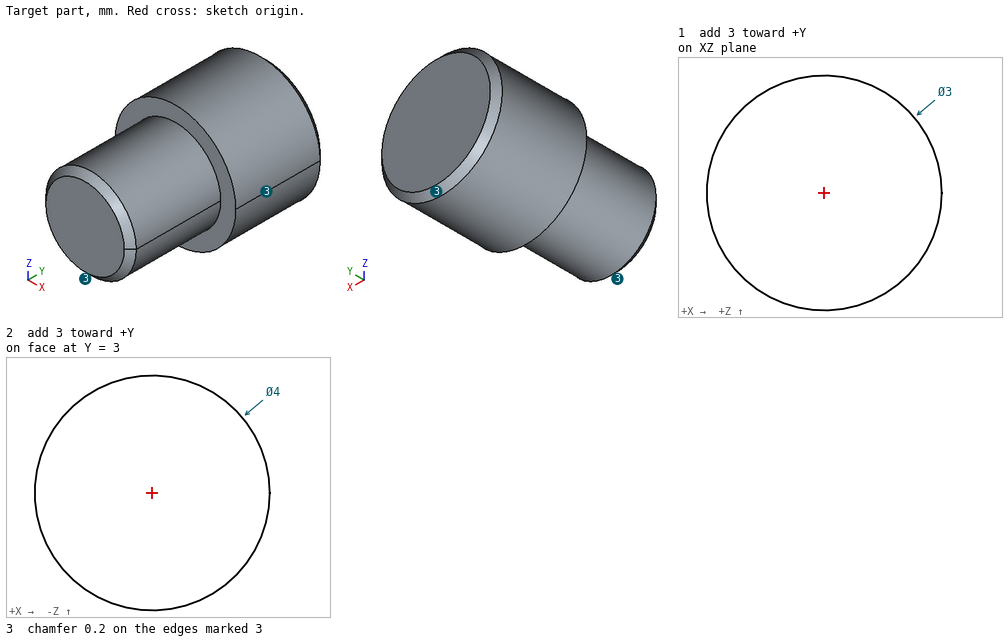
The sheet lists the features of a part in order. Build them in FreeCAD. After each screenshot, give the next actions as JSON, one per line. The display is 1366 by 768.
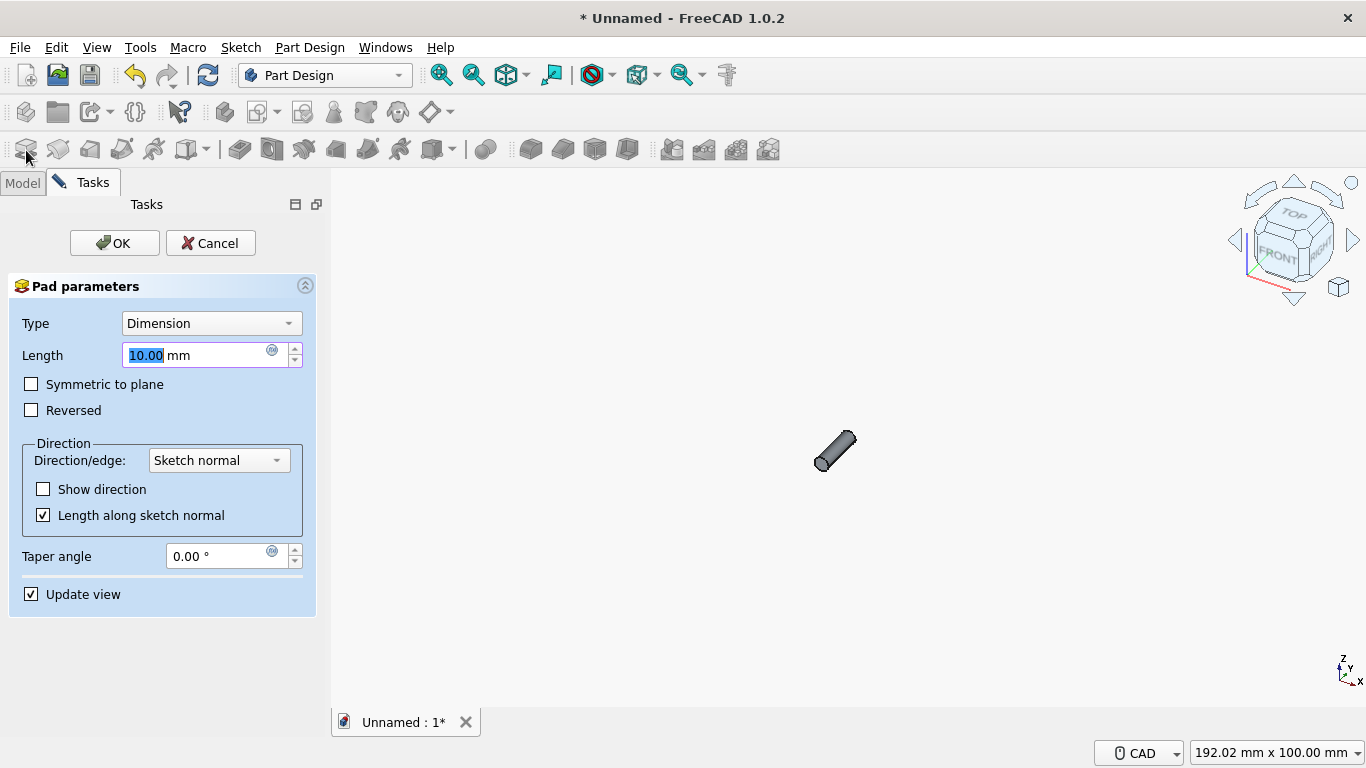
{"action": "type", "text": "3"}
{"action": "key", "text": "Tab"}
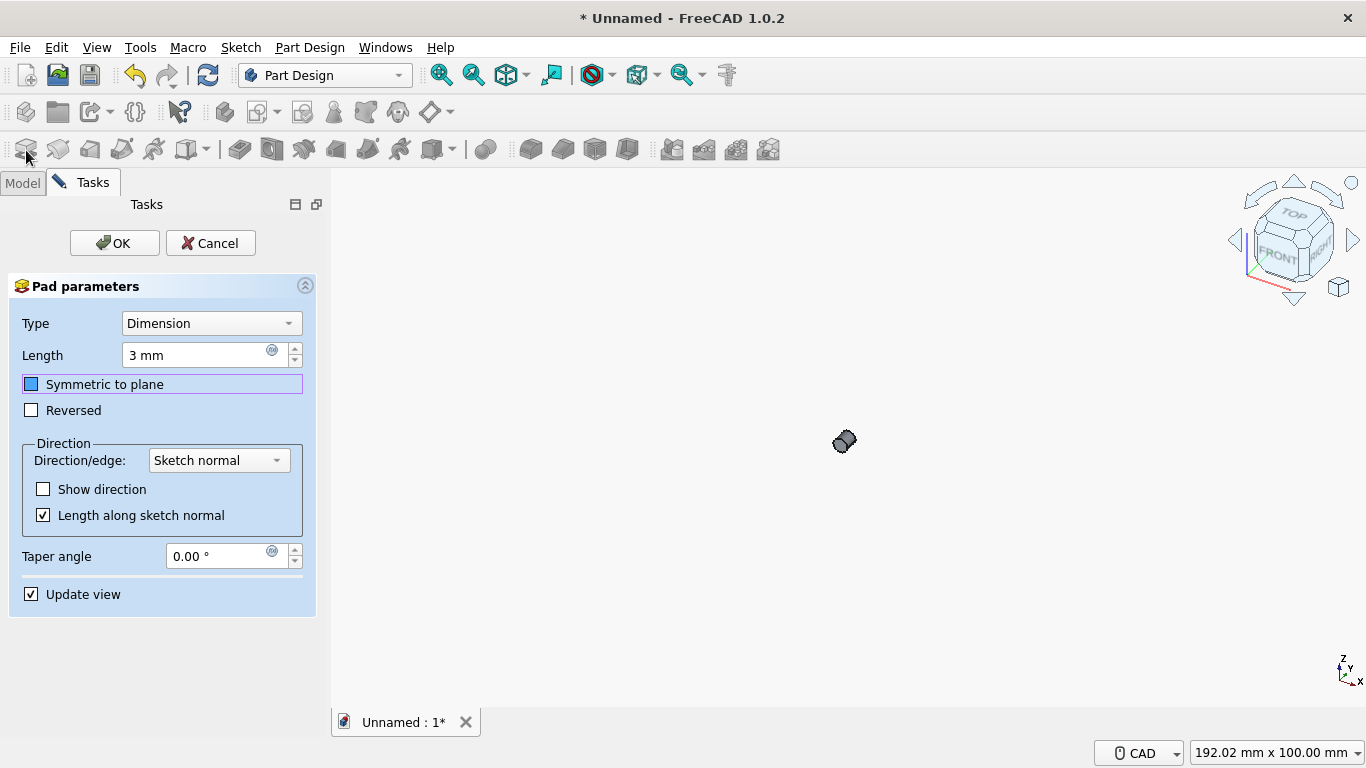
{"action": "left_click", "coordinate": [30, 410]}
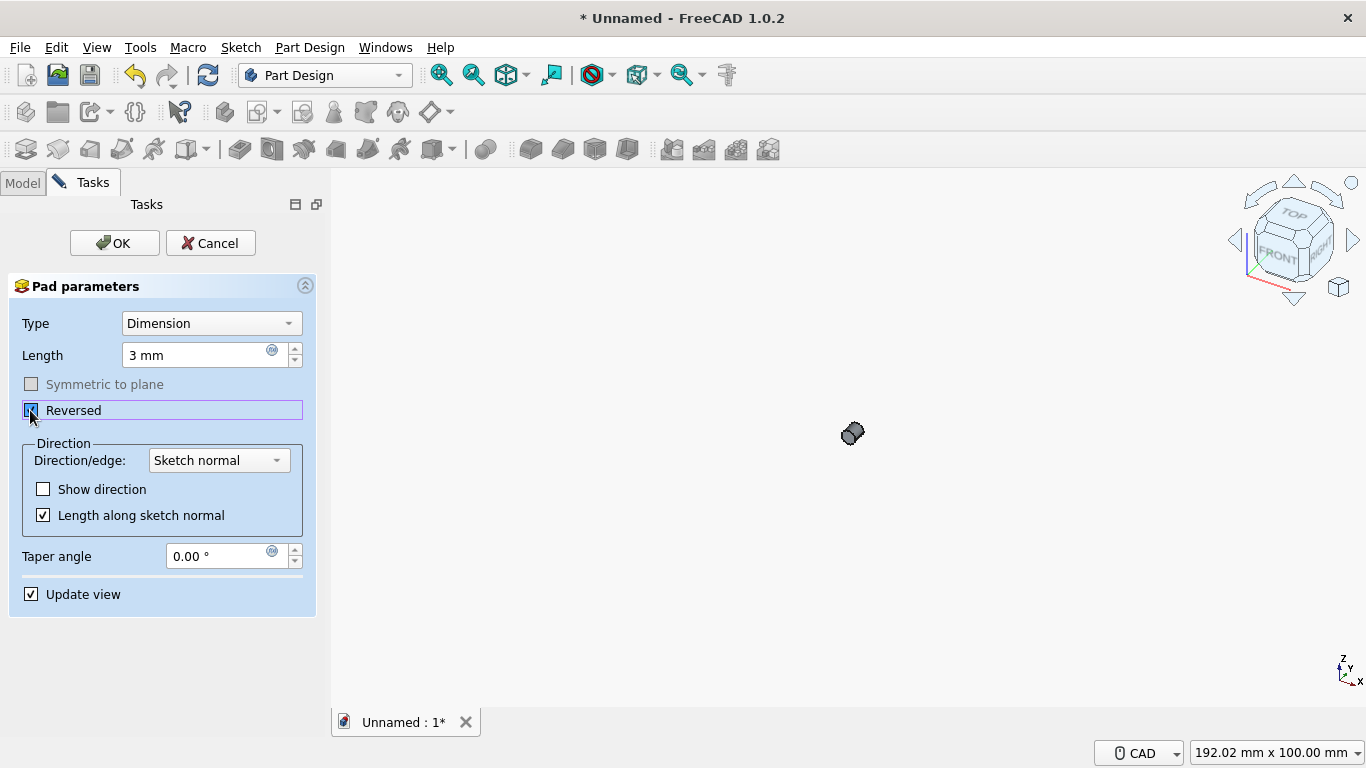
{"action": "left_click", "coordinate": [115, 243]}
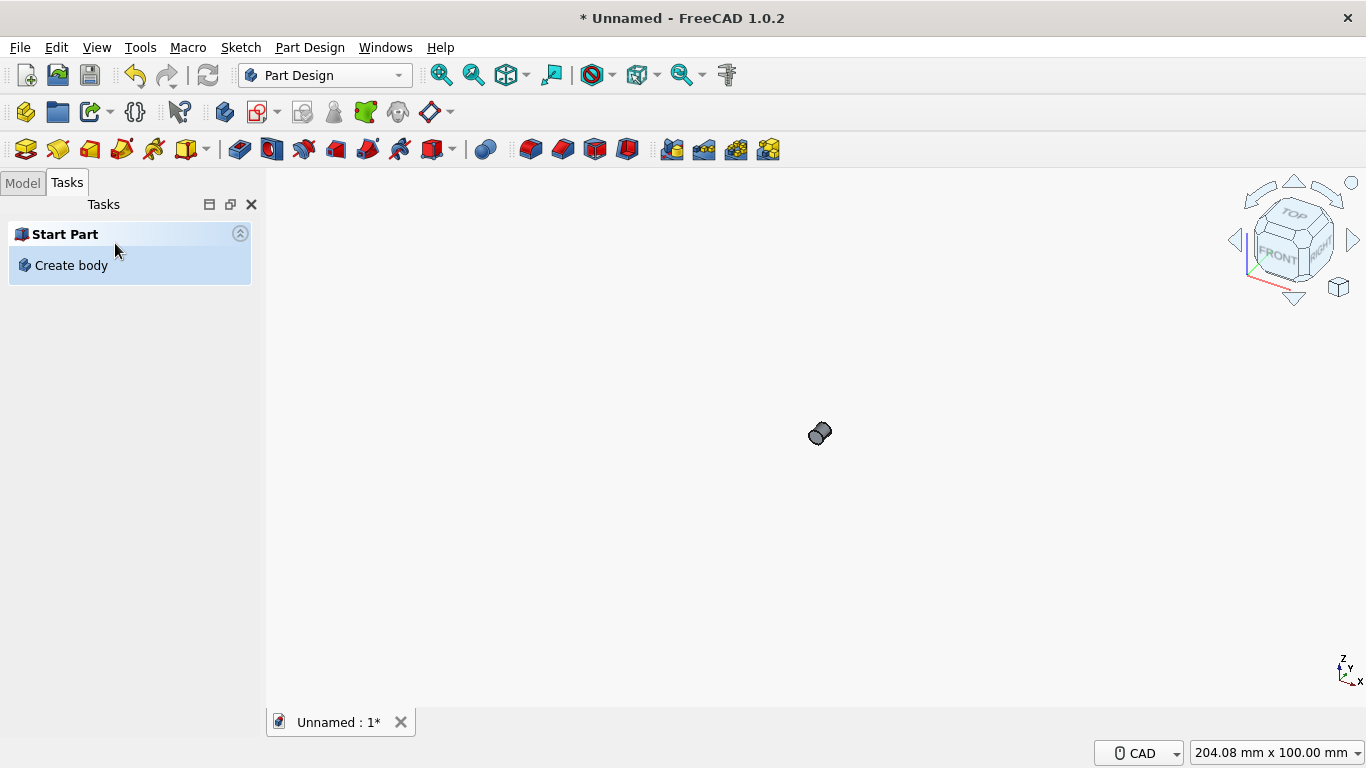
{"action": "left_click", "coordinate": [442, 76]}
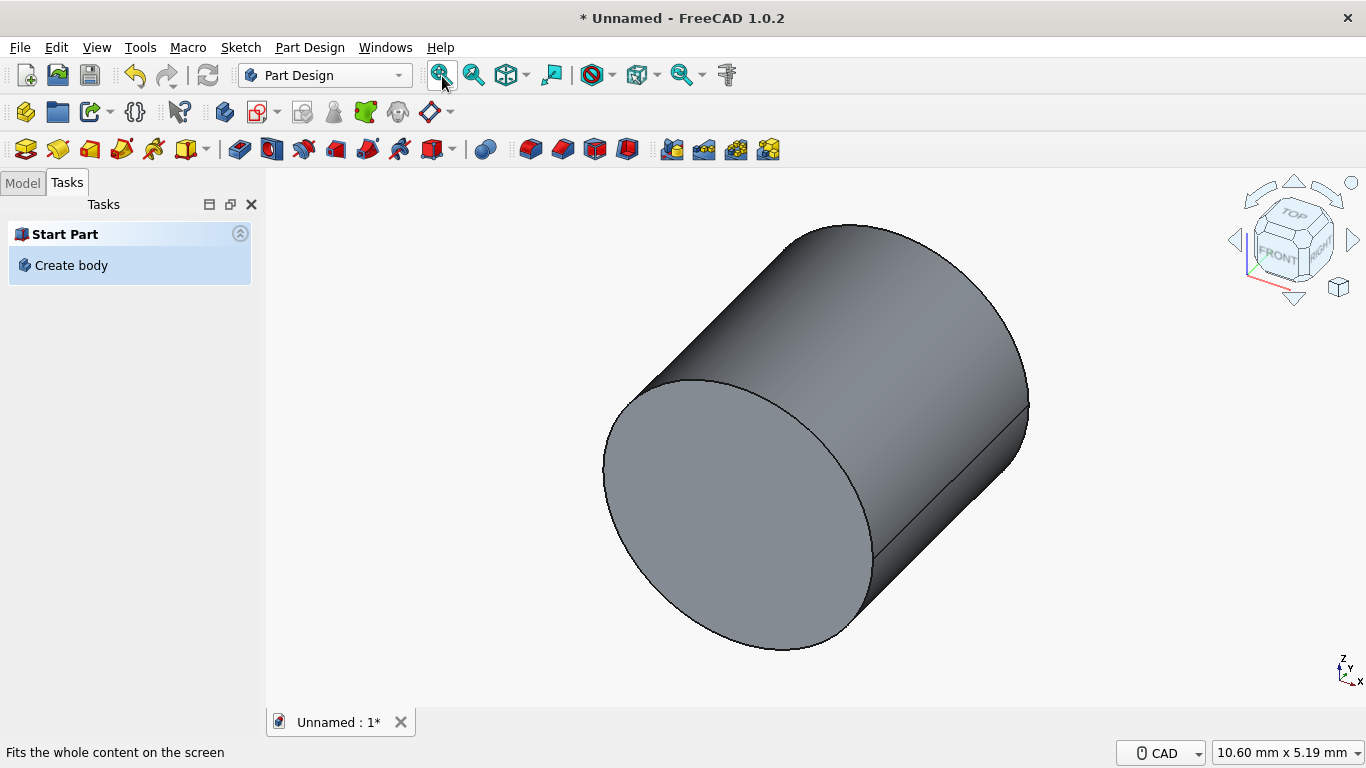
{"action": "key", "text": "4"}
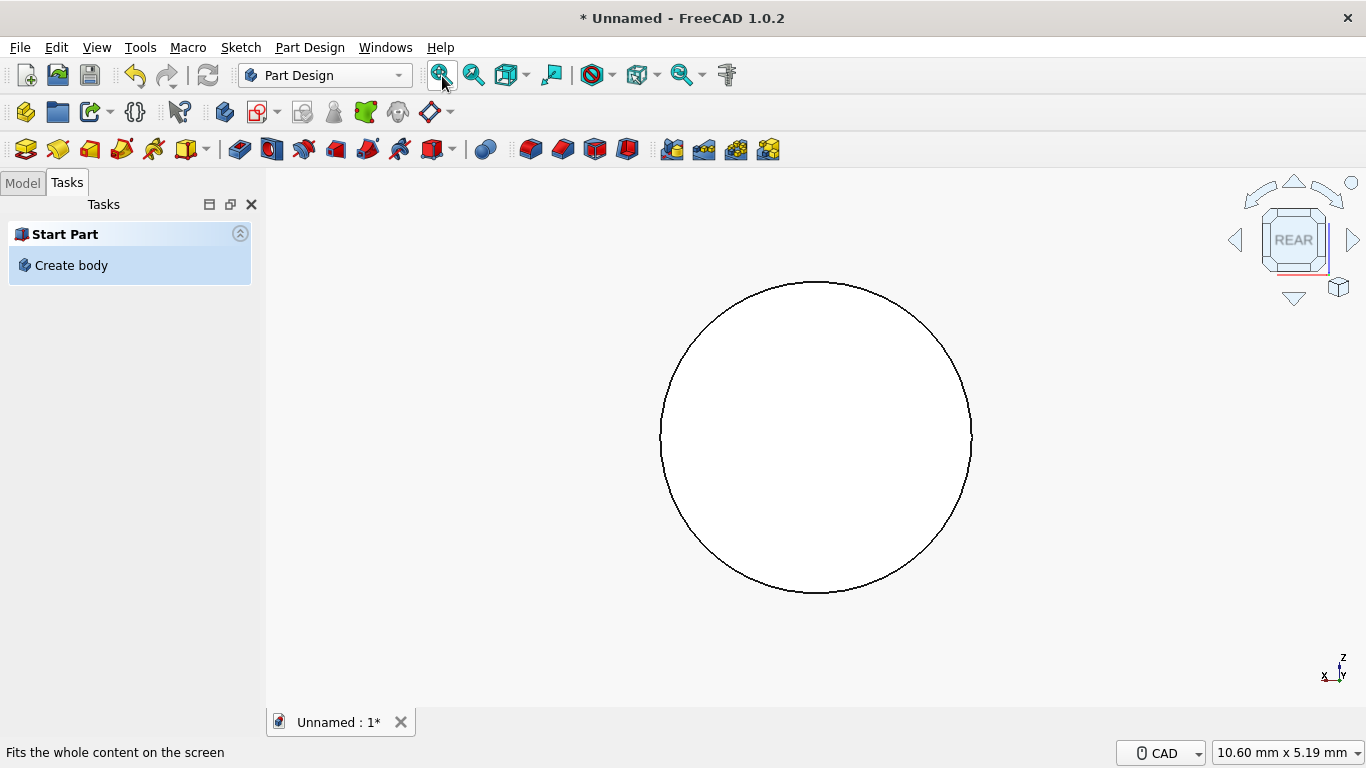
{"action": "left_click", "coordinate": [816, 437]}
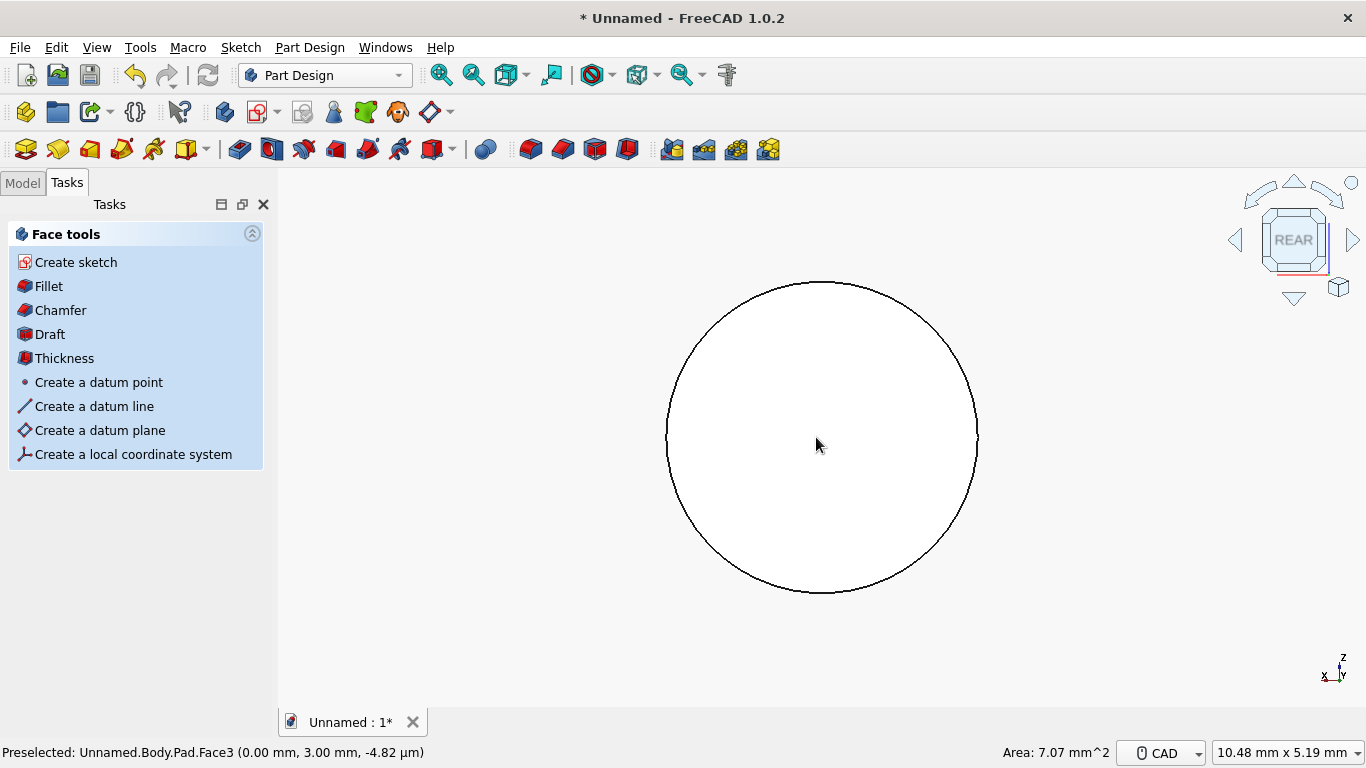
{"action": "left_click", "coordinate": [258, 112]}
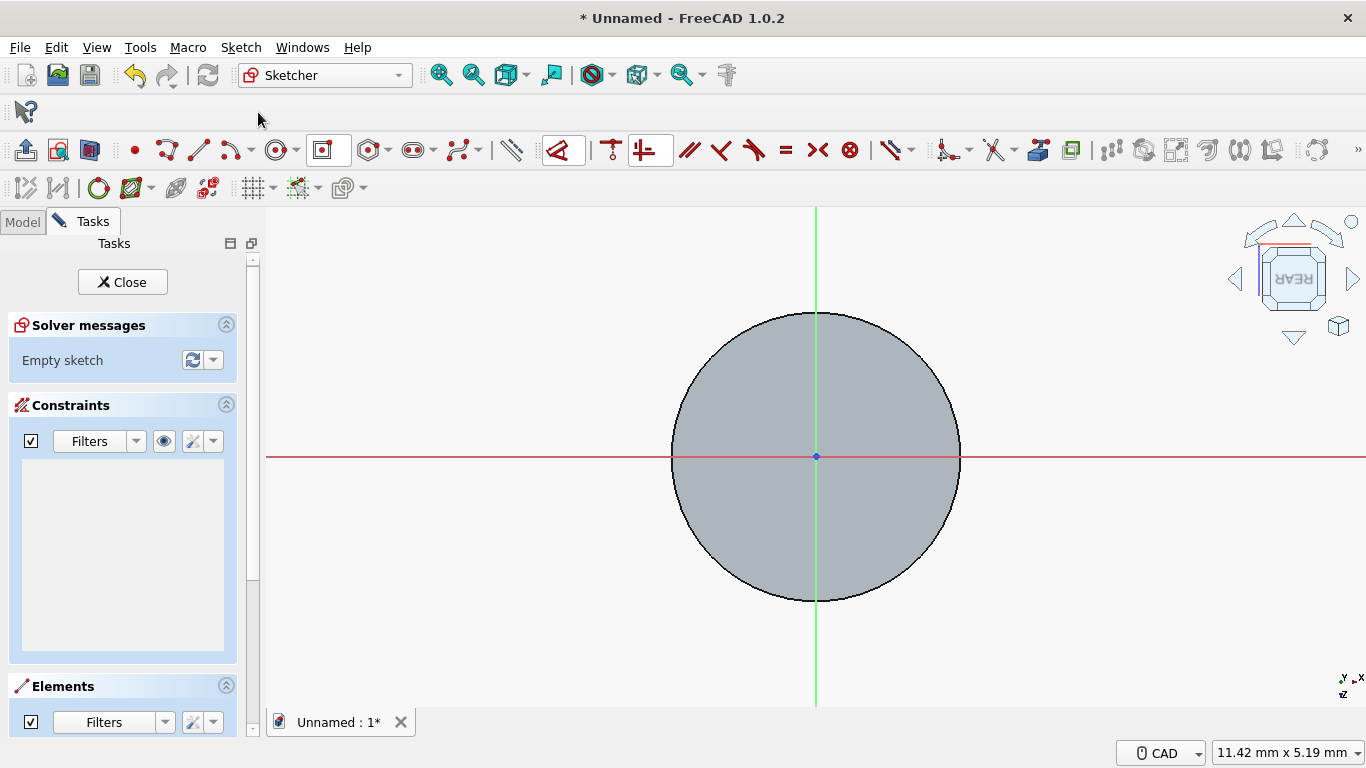
{"action": "key", "text": "g c"}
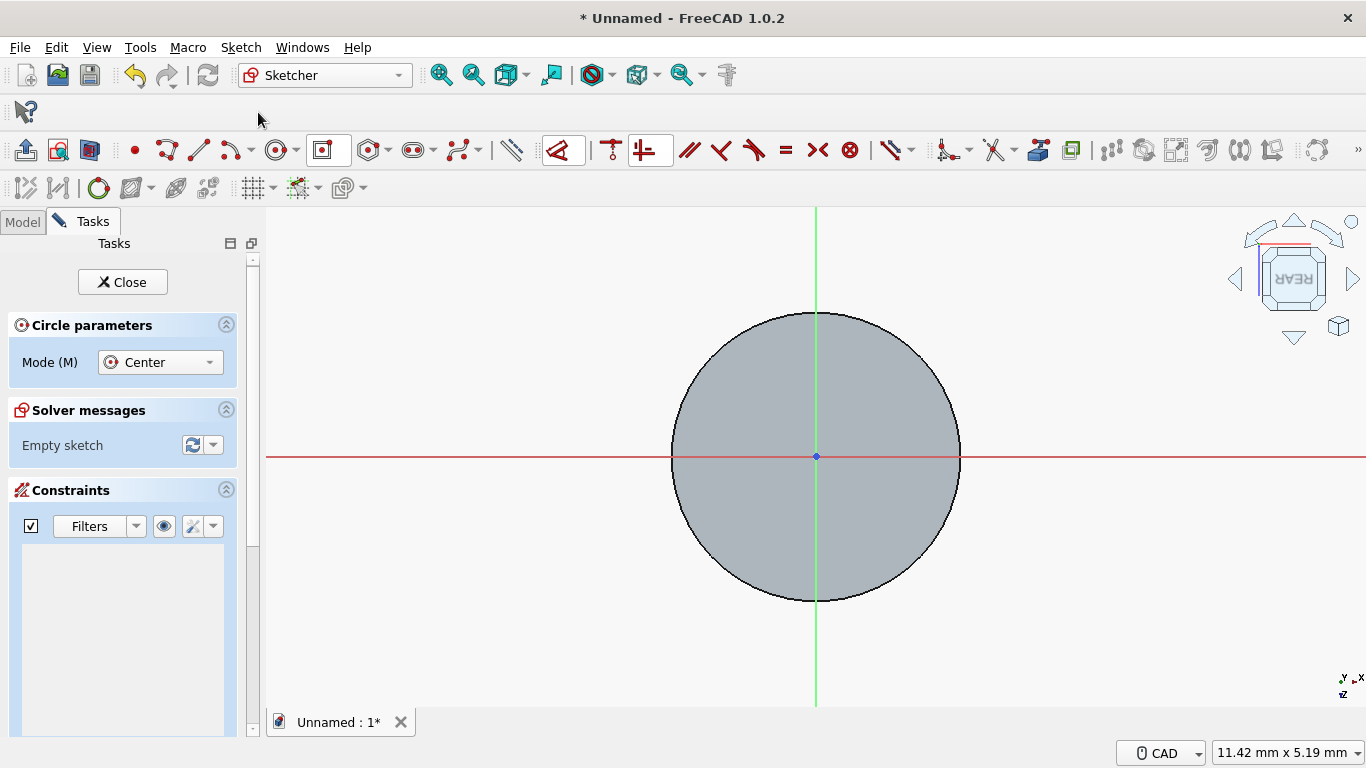
{"action": "left_click", "coordinate": [816, 457]}
{"action": "mouse_move", "coordinate": [952, 321]}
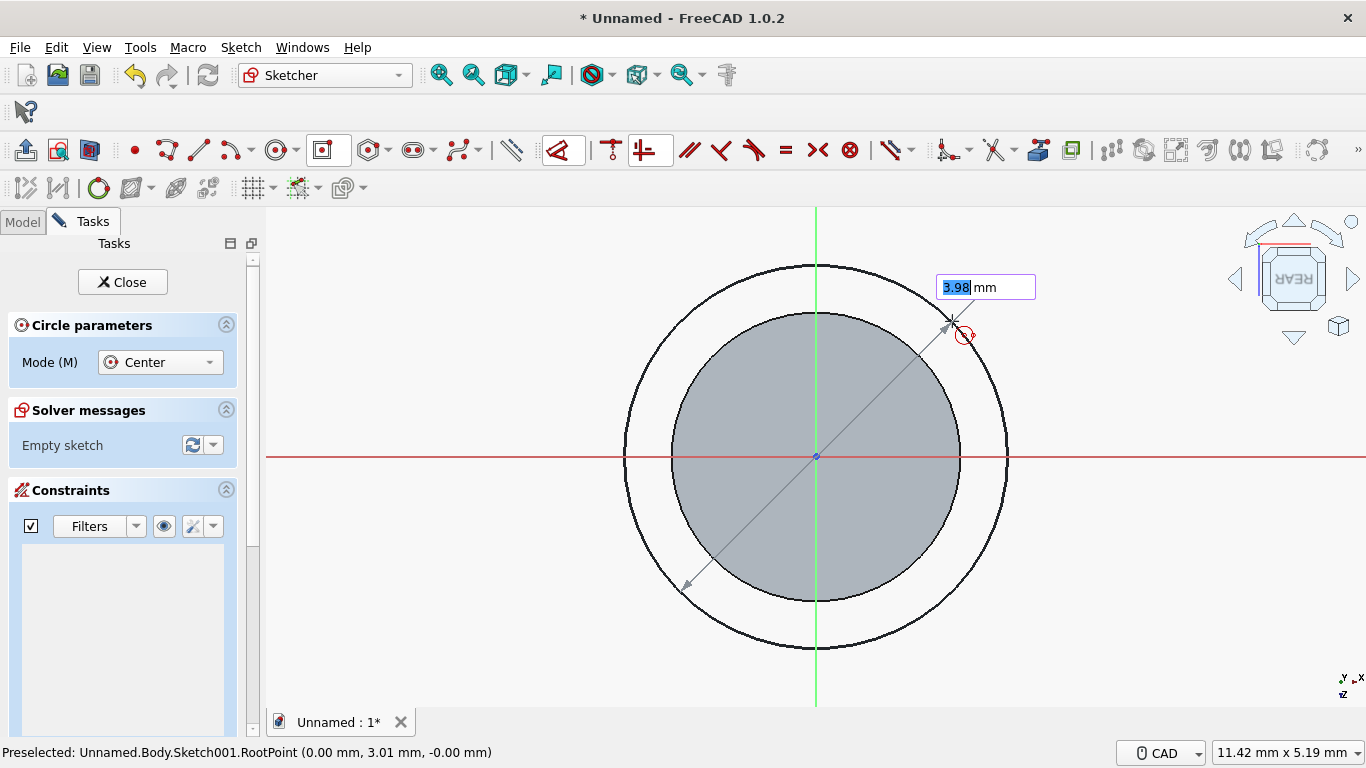
{"action": "type", "text": "4"}
{"action": "key", "text": "Return"}
{"action": "key", "text": "Escape"}